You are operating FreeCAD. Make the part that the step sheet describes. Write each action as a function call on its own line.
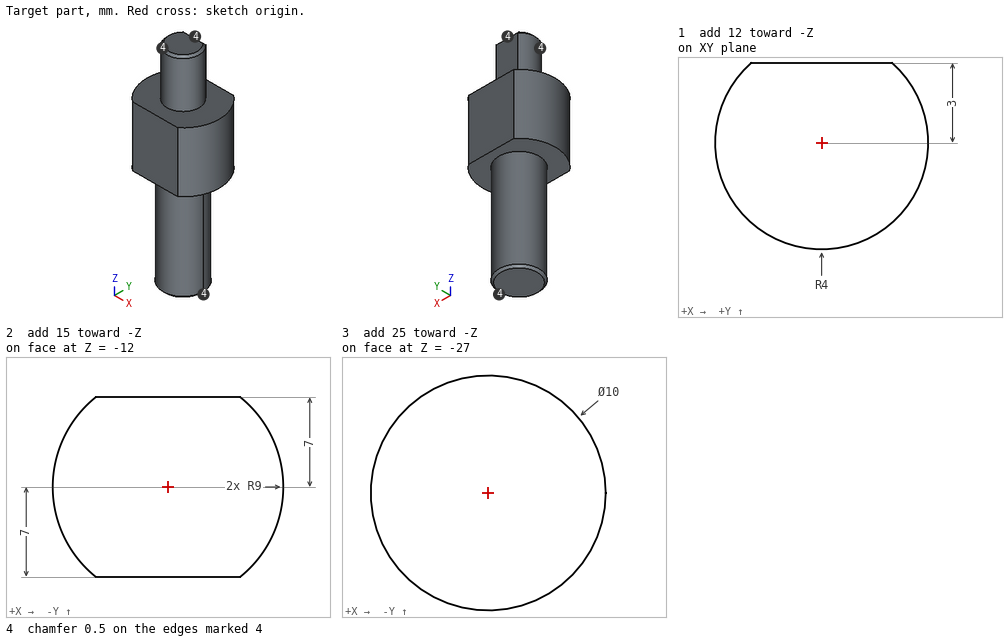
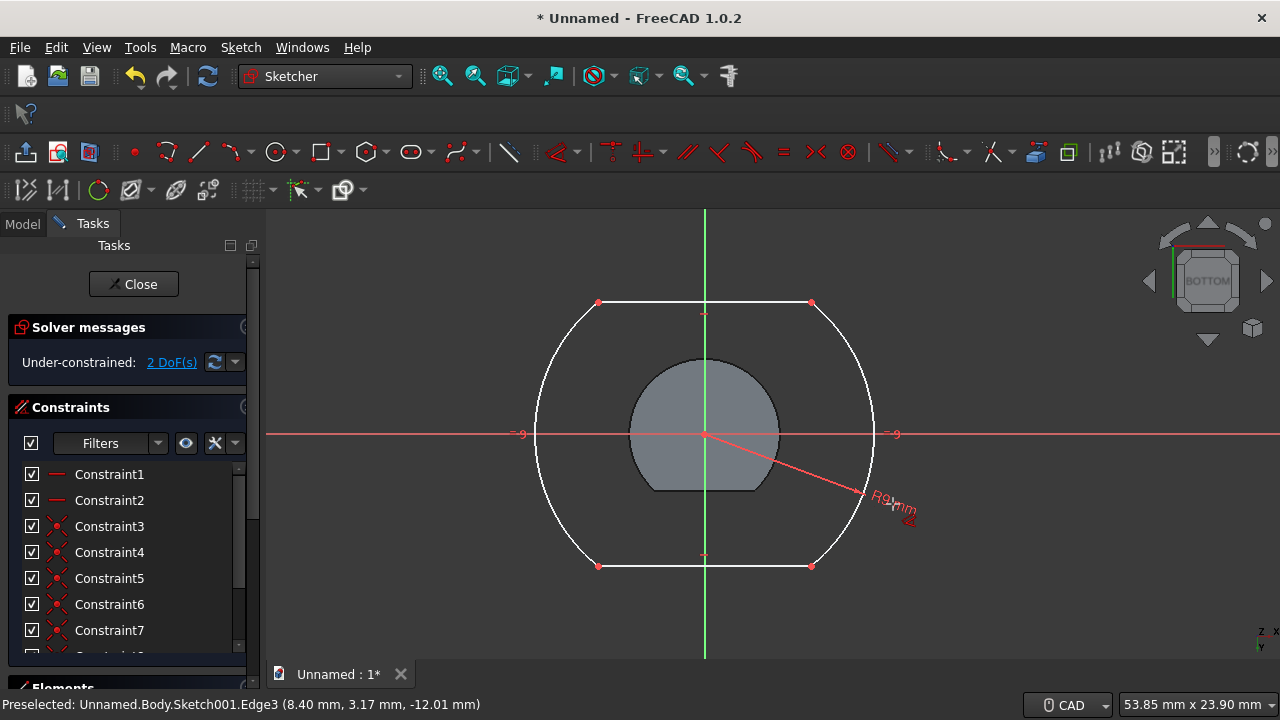
click(598, 566)
click(564, 500)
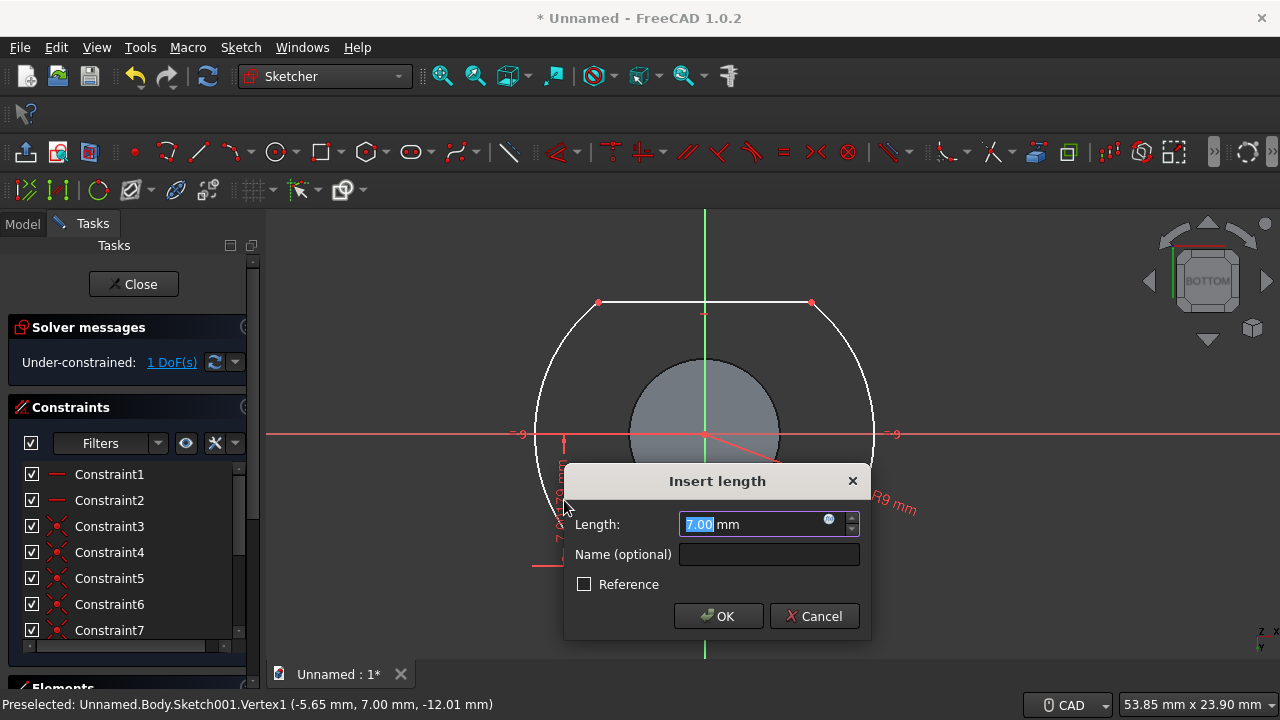
text(7)
key(Return)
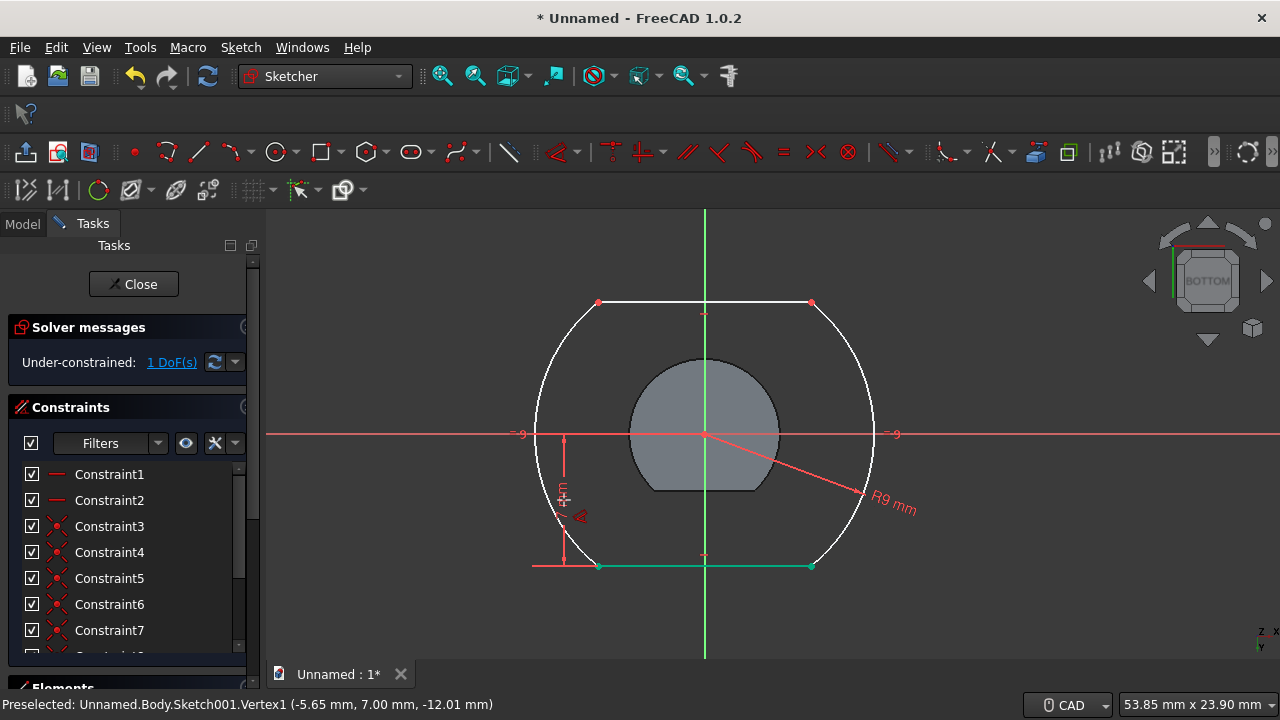
click(811, 302)
click(845, 368)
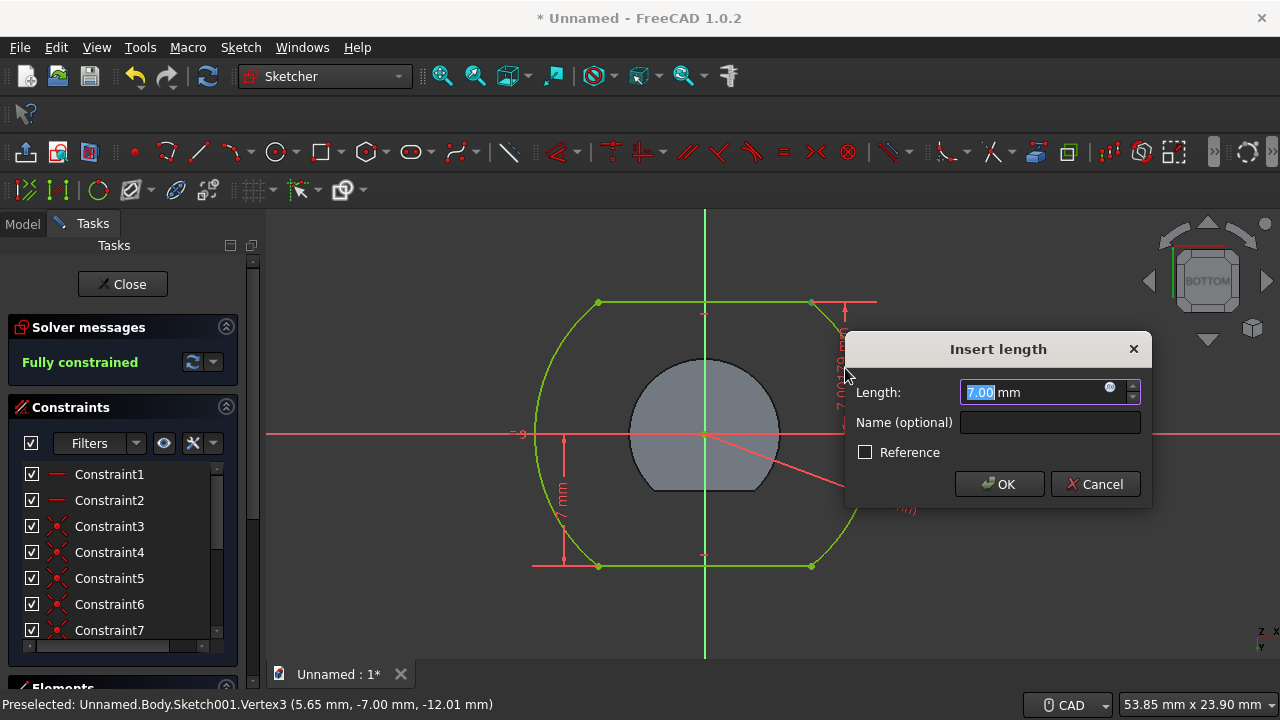
text(7)
key(Return)
key(Escape)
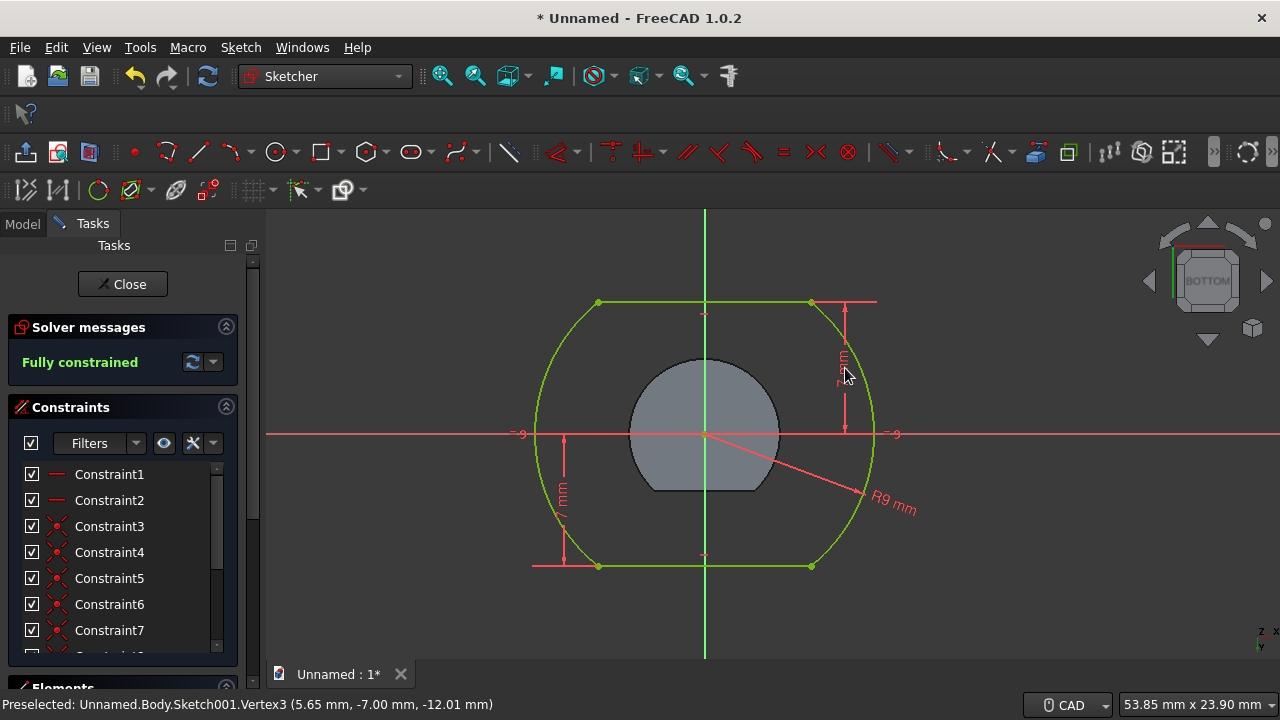
click(123, 284)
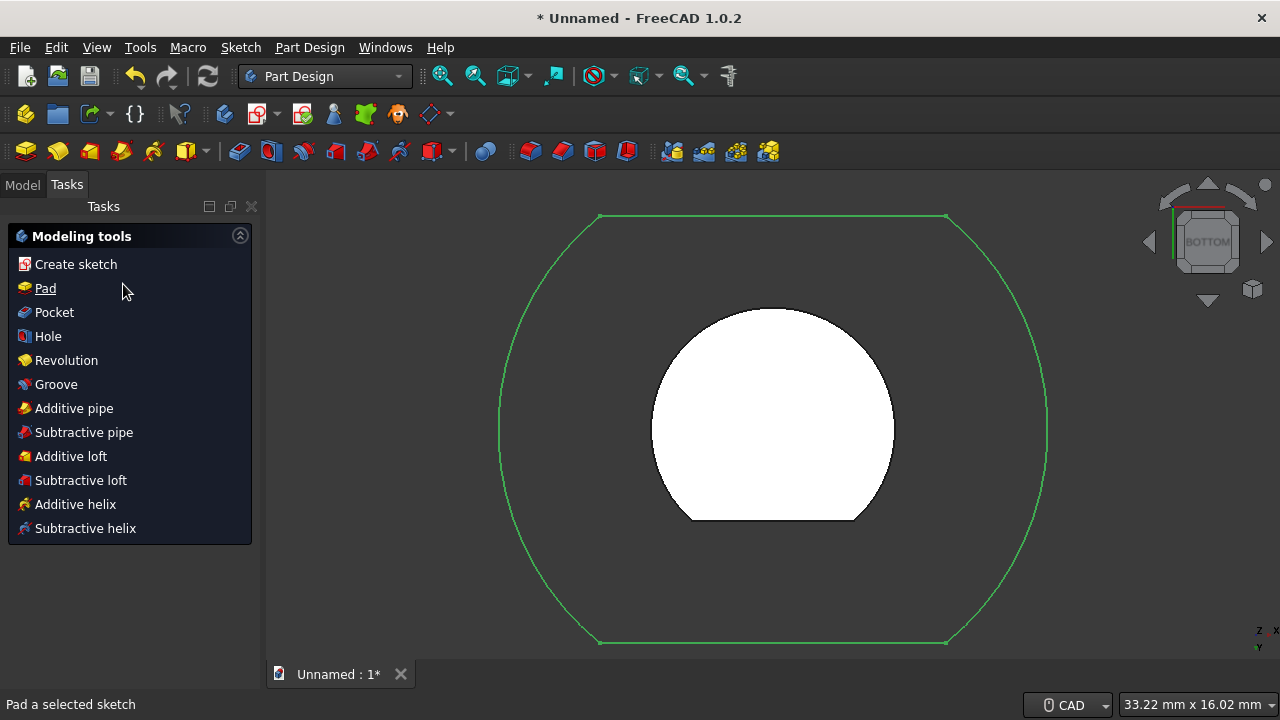
click(26, 152)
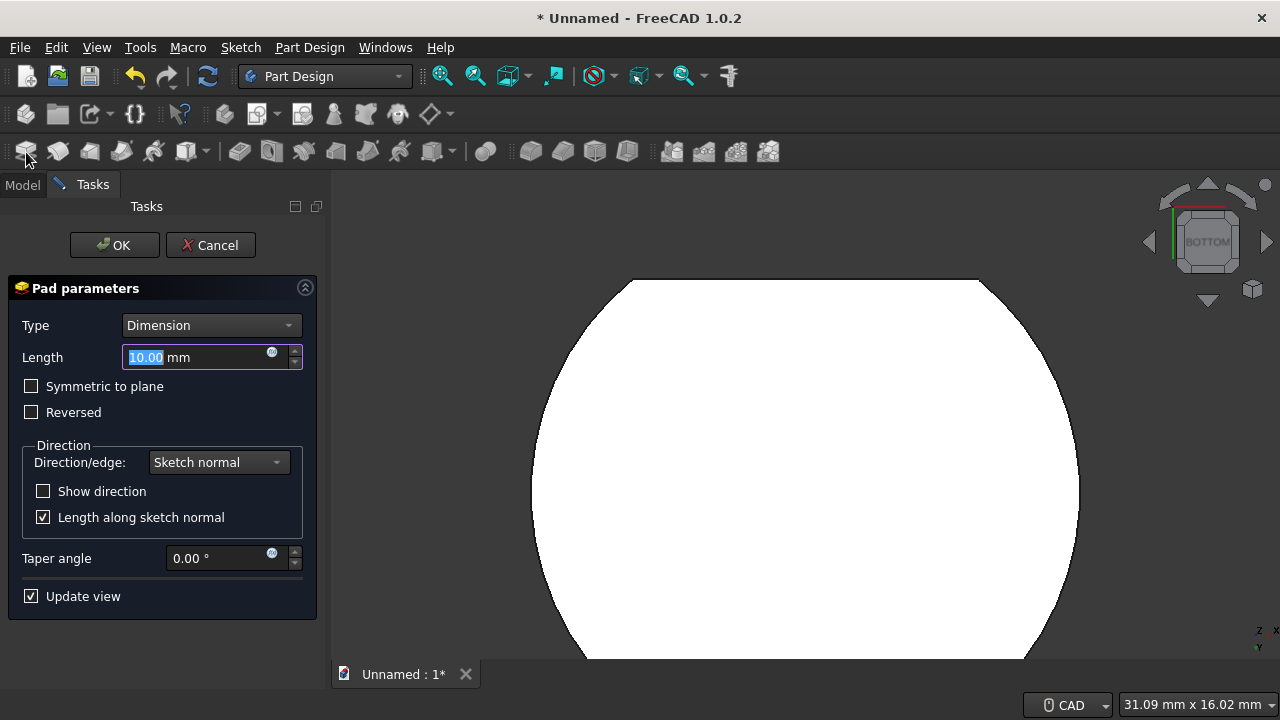
text(15)
key(Tab)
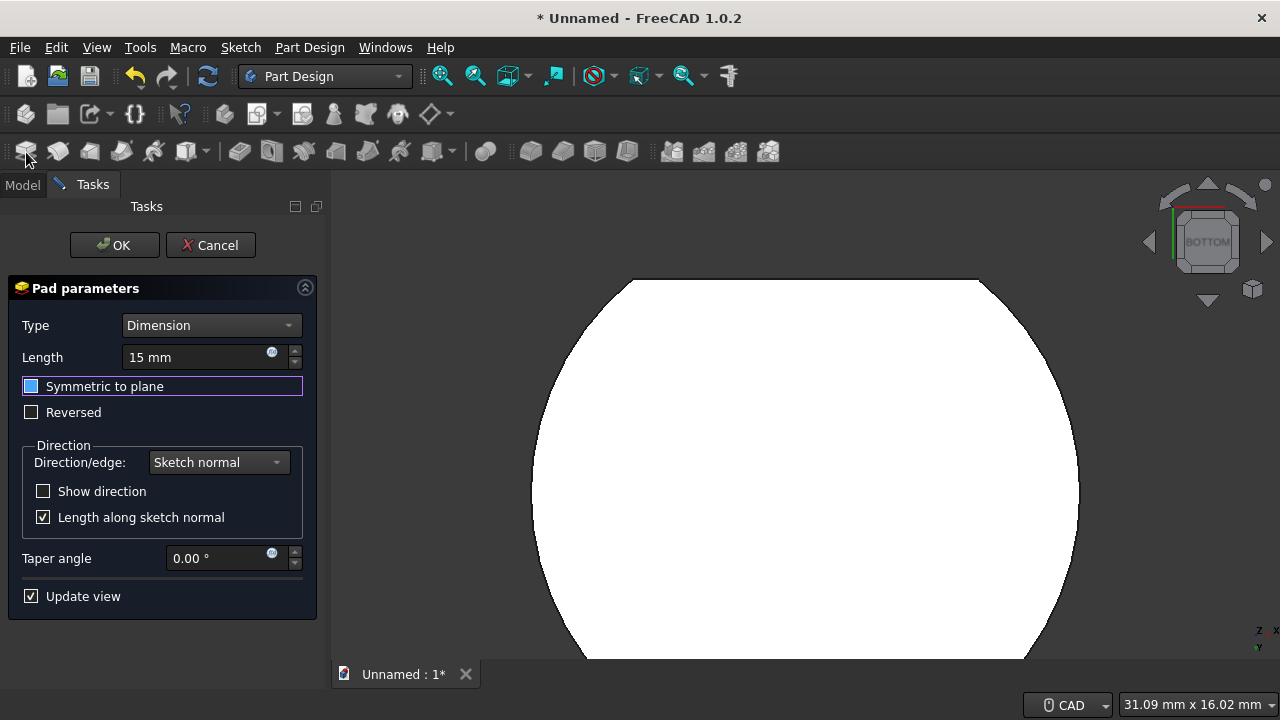
click(115, 245)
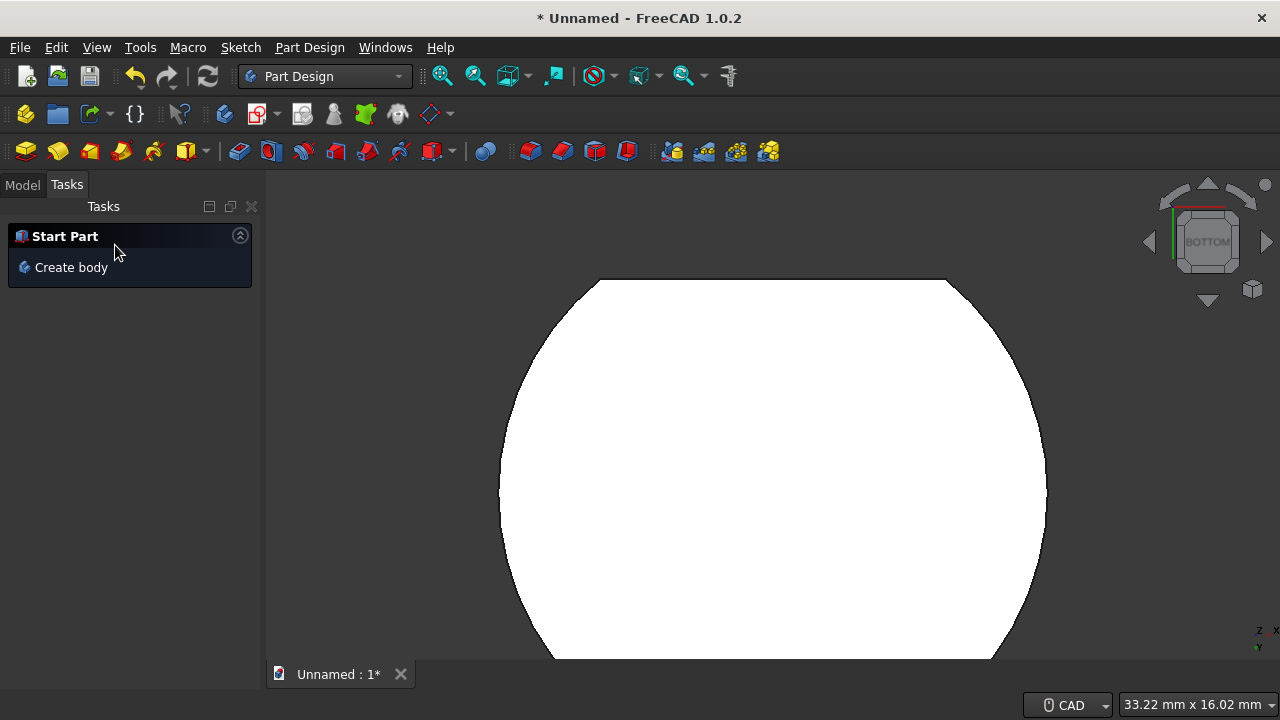
key(v)
key(f)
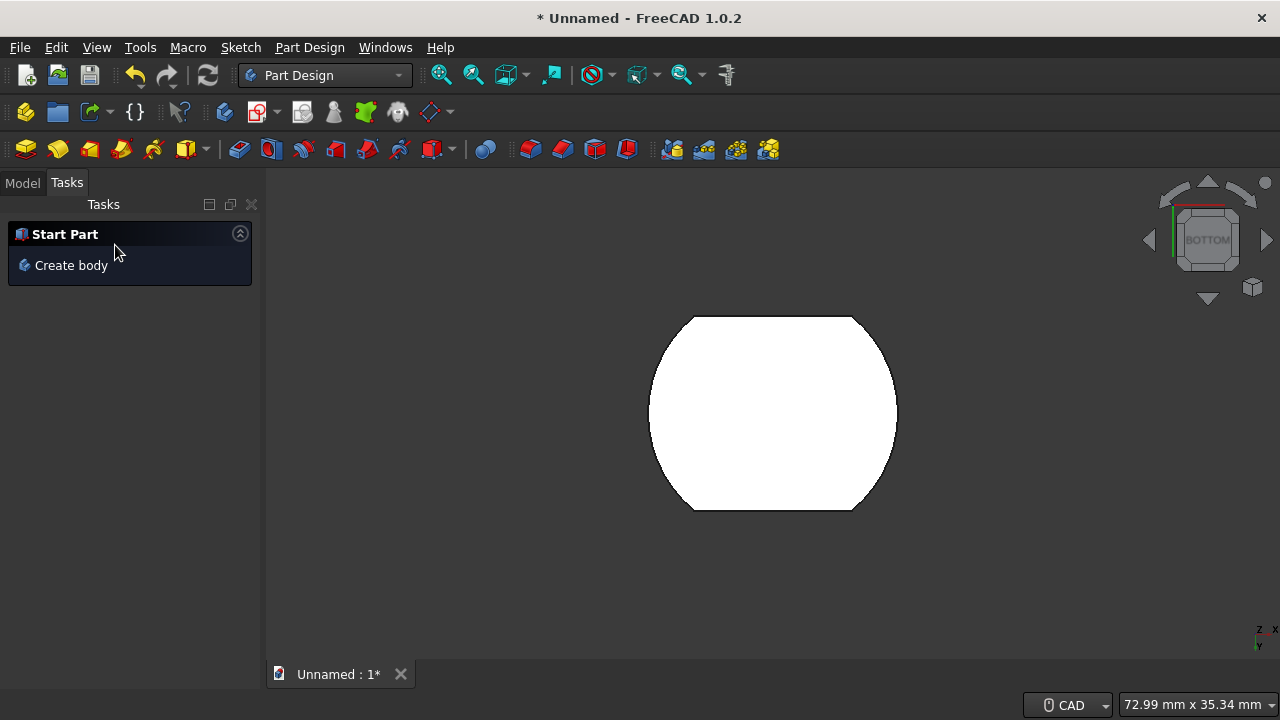
click(773, 412)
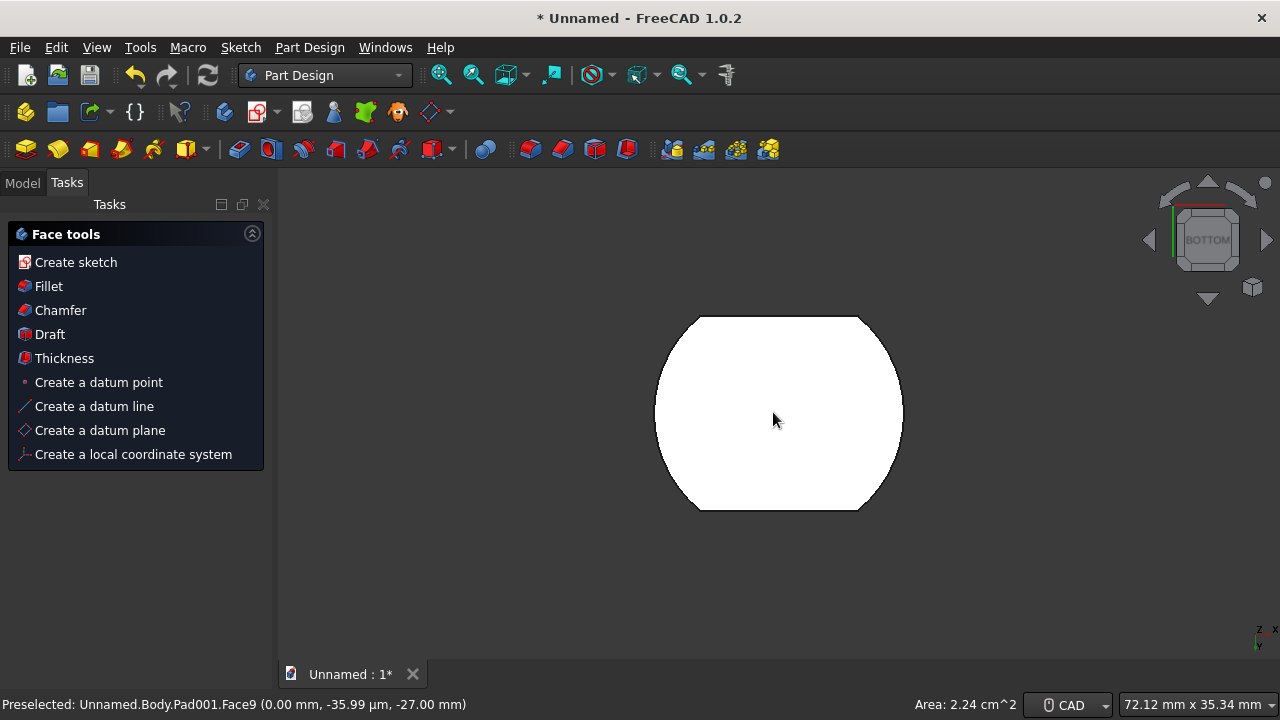
click(258, 112)